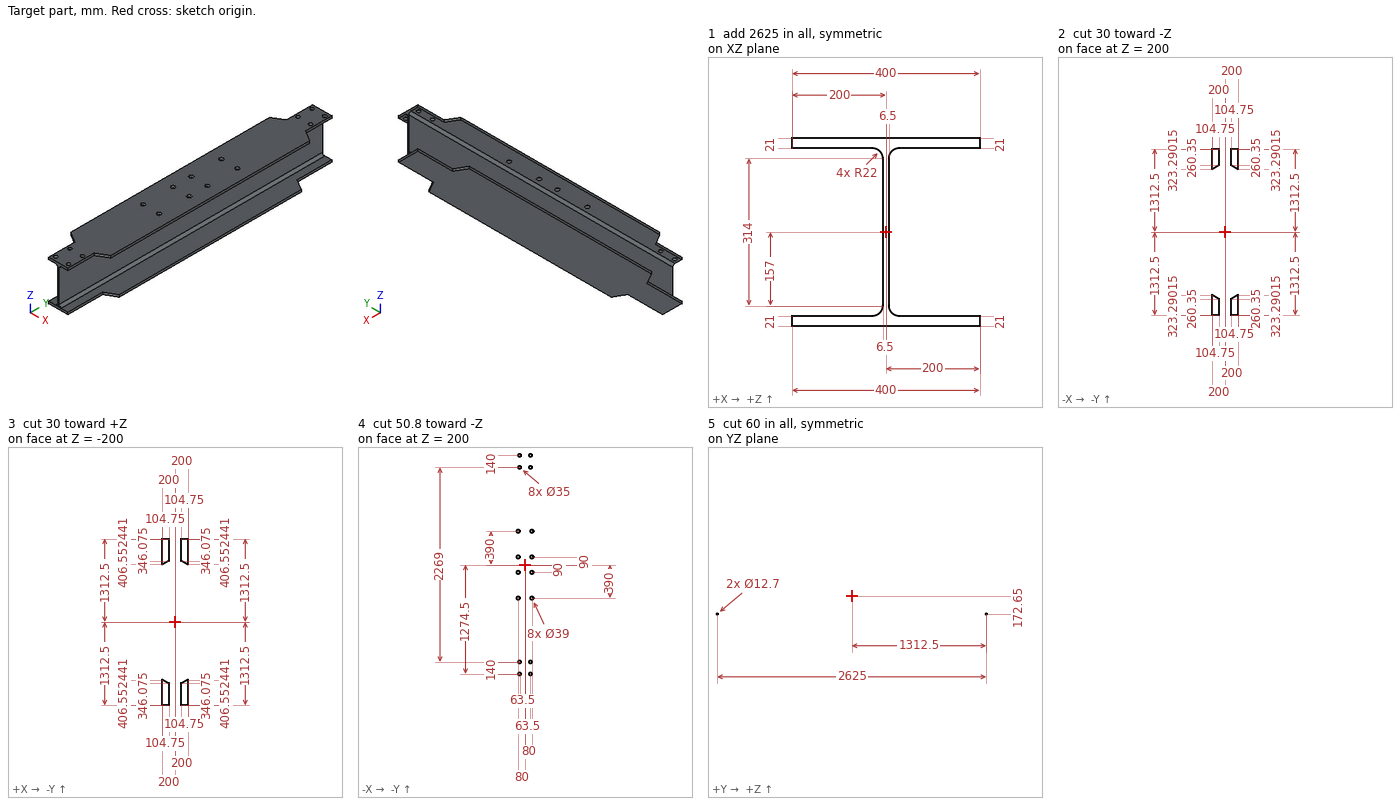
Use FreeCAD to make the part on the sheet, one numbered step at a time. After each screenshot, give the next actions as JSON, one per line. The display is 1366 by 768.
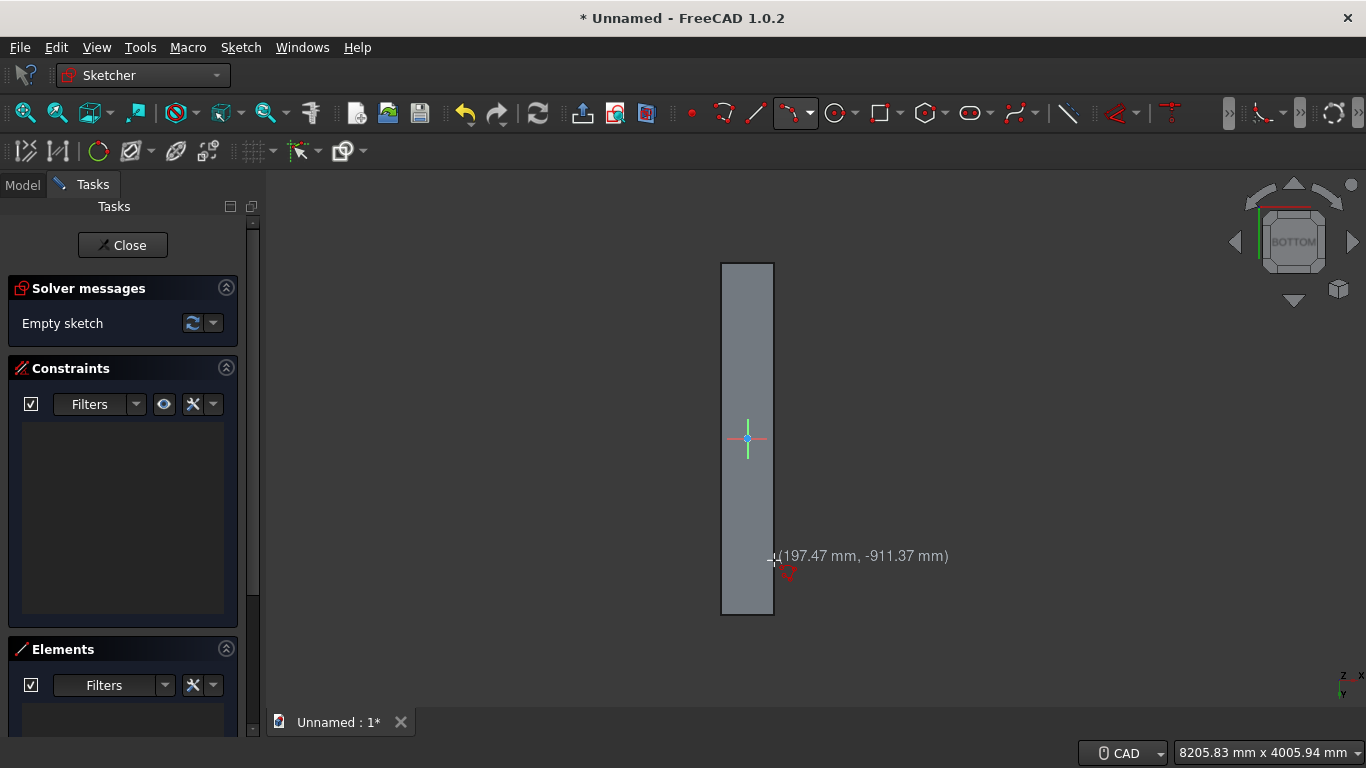
{"action": "scroll", "coordinate": [760, 568], "scroll_direction": "up", "scroll_amount": 2}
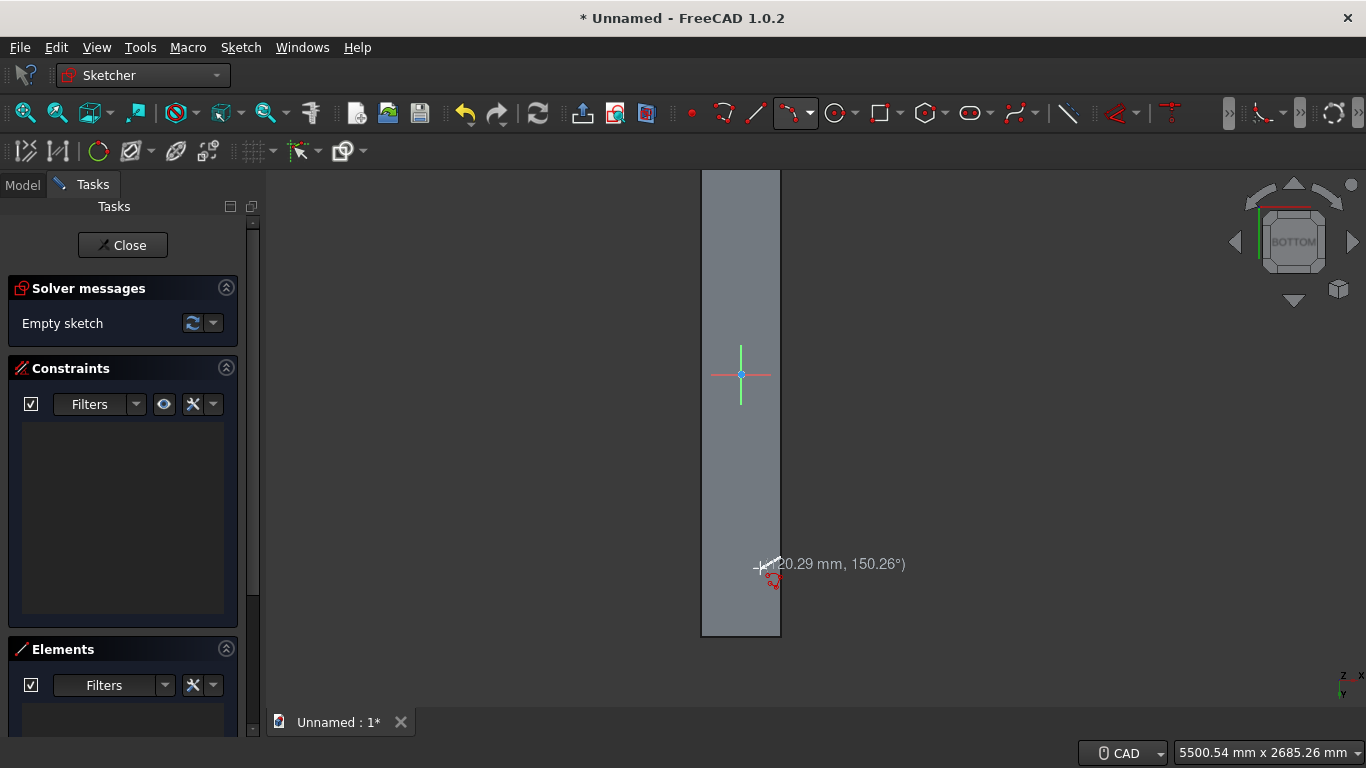
{"action": "left_click", "coordinate": [760, 568]}
{"action": "left_click", "coordinate": [760, 637]}
{"action": "left_click", "coordinate": [781, 637]}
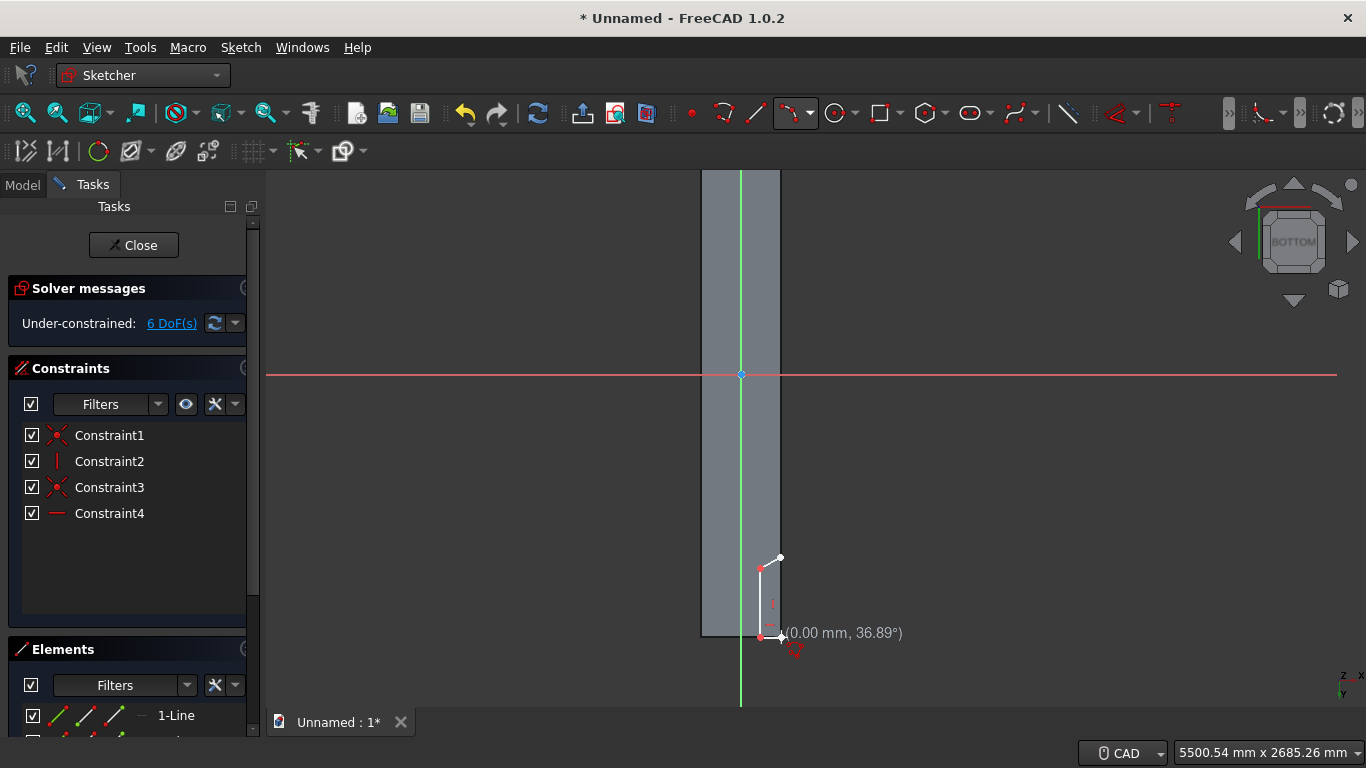
{"action": "scroll", "coordinate": [781, 556], "scroll_direction": "up", "scroll_amount": 2}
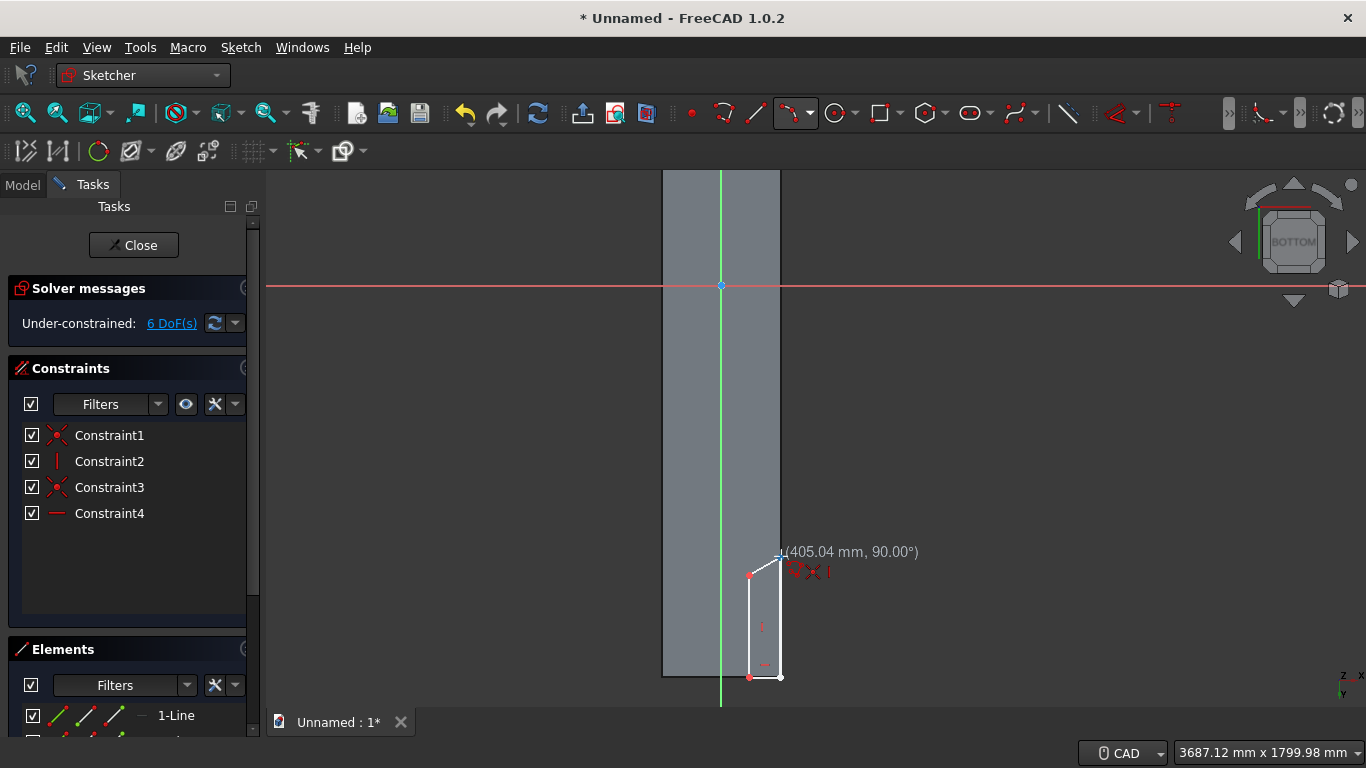
{"action": "left_click", "coordinate": [780, 557]}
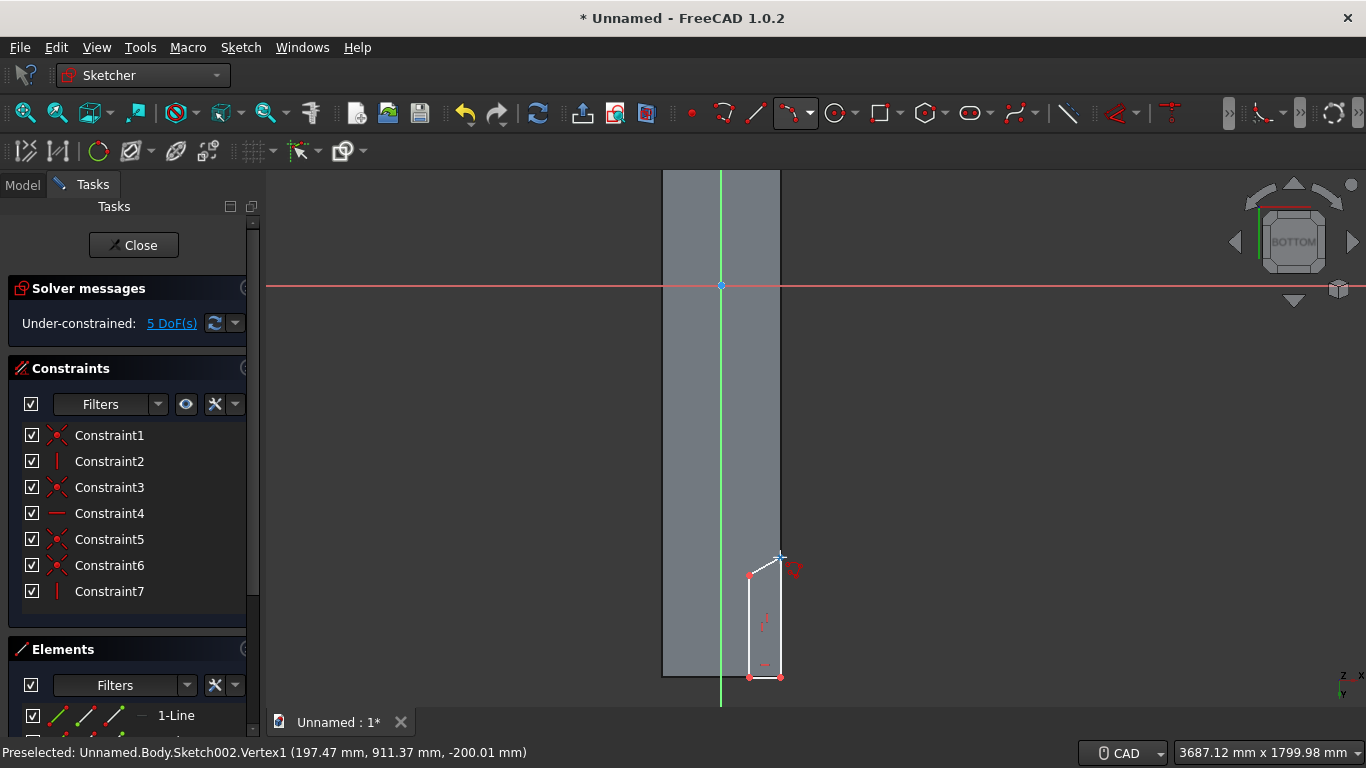
{"action": "left_click", "coordinate": [662, 556]}
{"action": "left_click", "coordinate": [662, 677]}
{"action": "left_click", "coordinate": [693, 677]}
{"action": "left_click", "coordinate": [693, 574]}
{"action": "left_click", "coordinate": [662, 557]}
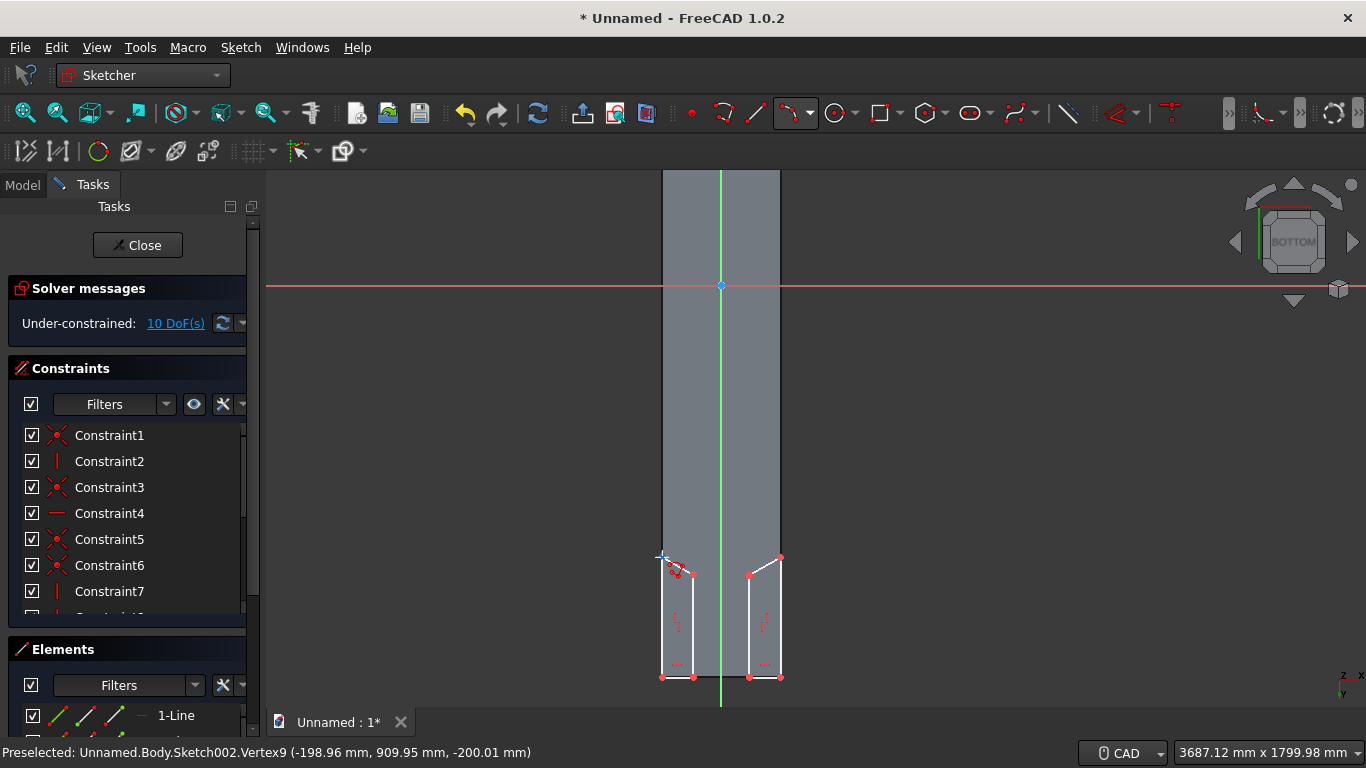
{"action": "scroll", "coordinate": [769, 563], "scroll_direction": "down", "scroll_amount": 4}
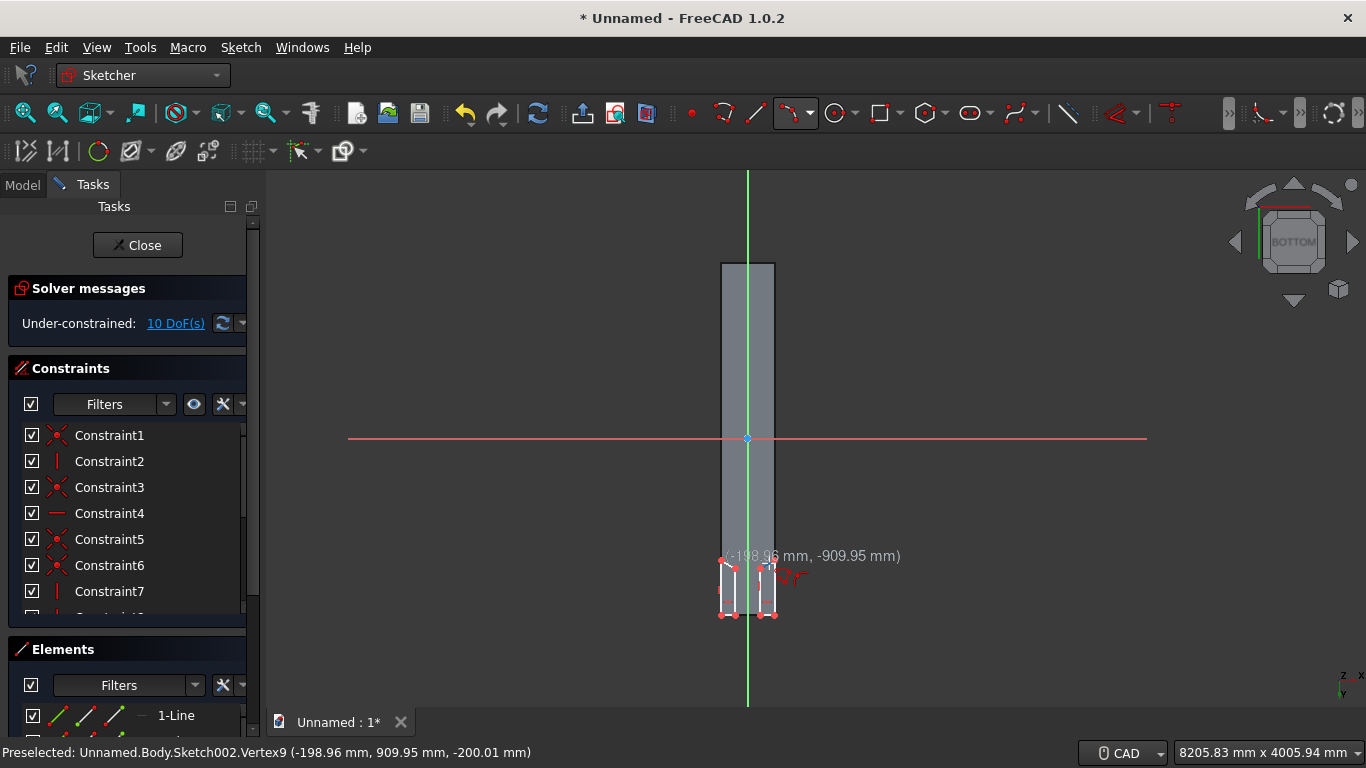
{"action": "left_click", "coordinate": [721, 317]}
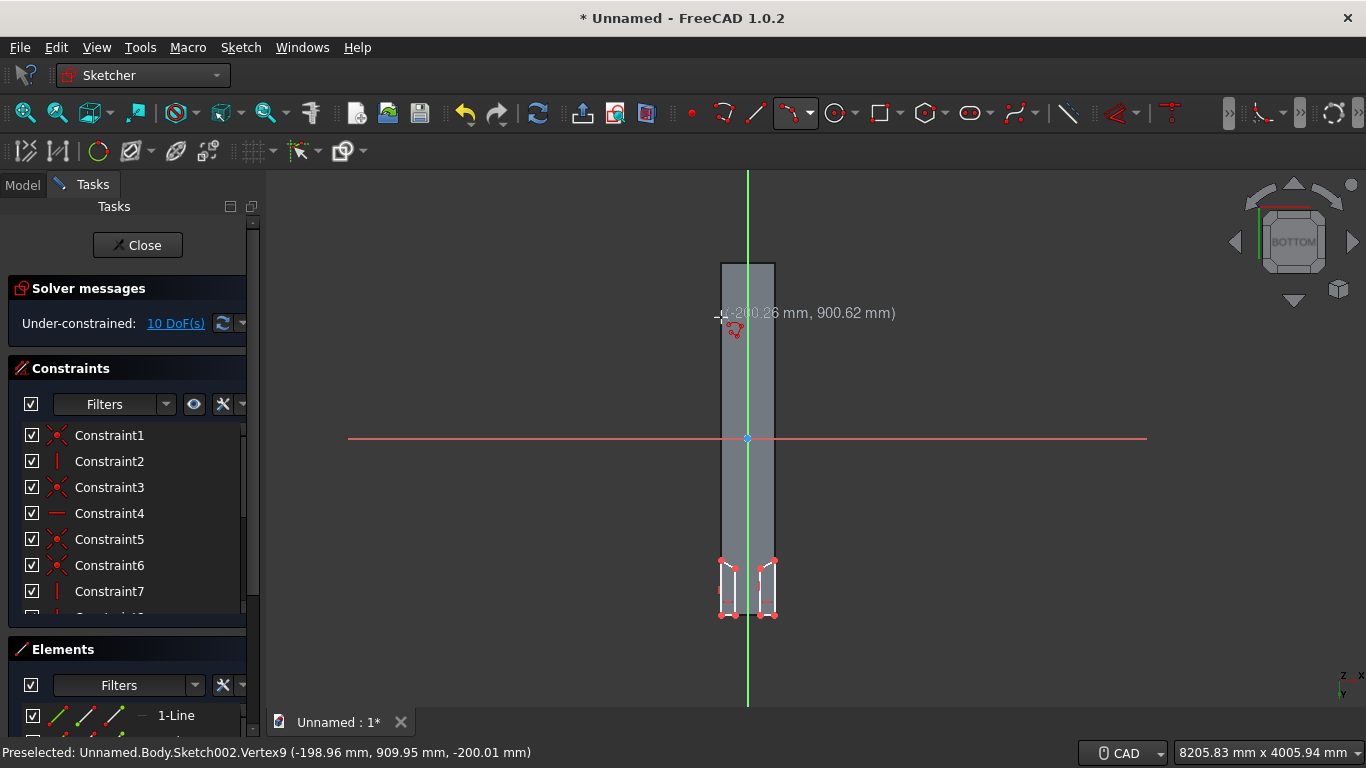
{"action": "scroll", "coordinate": [735, 309], "scroll_direction": "up", "scroll_amount": 2}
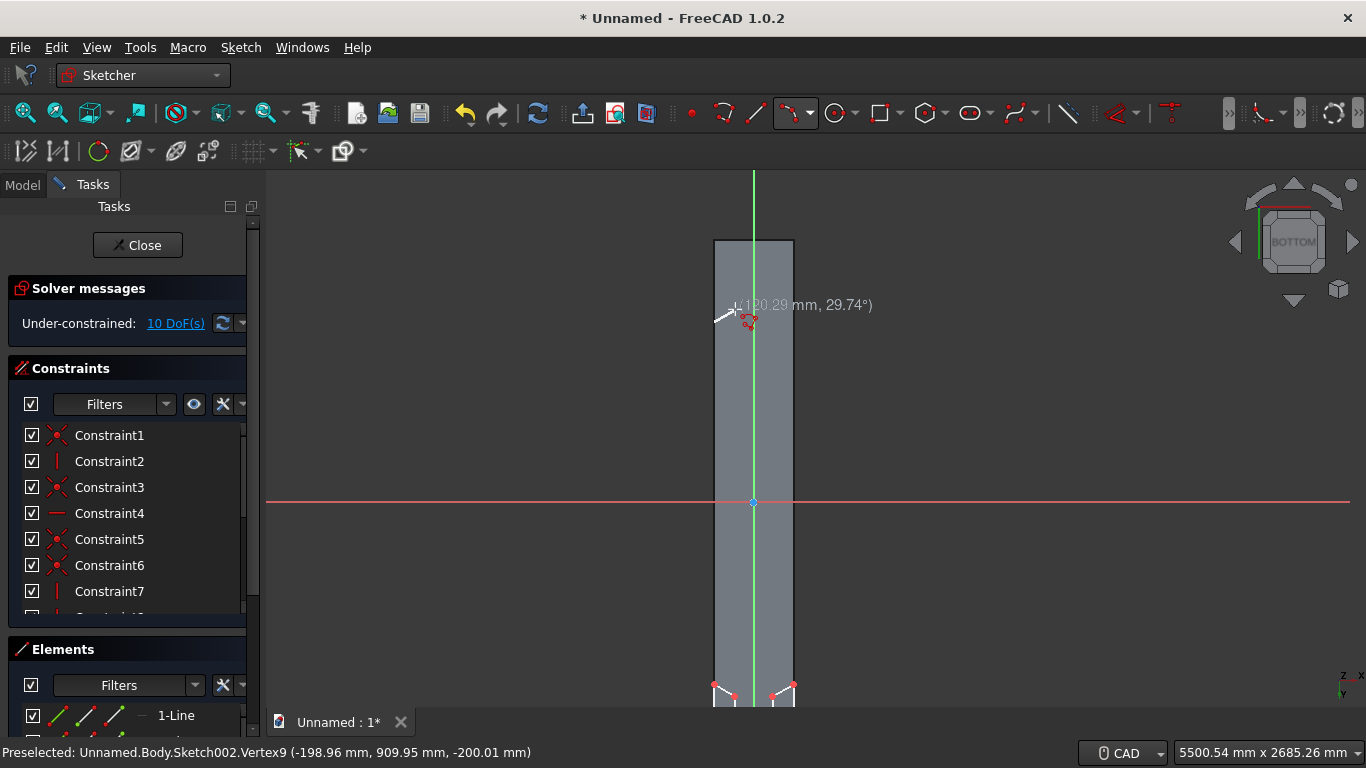
{"action": "left_click", "coordinate": [735, 309]}
{"action": "left_click", "coordinate": [735, 240]}
{"action": "left_click", "coordinate": [714, 240]}